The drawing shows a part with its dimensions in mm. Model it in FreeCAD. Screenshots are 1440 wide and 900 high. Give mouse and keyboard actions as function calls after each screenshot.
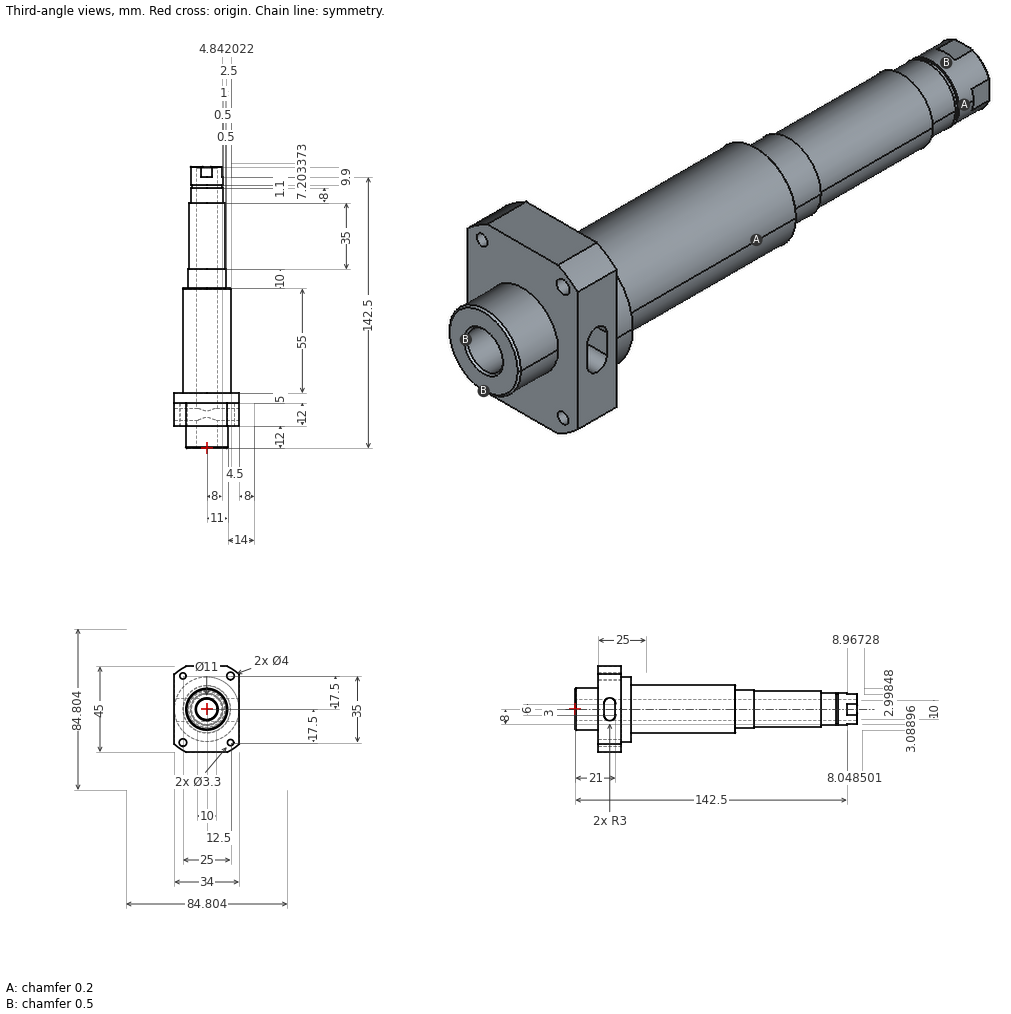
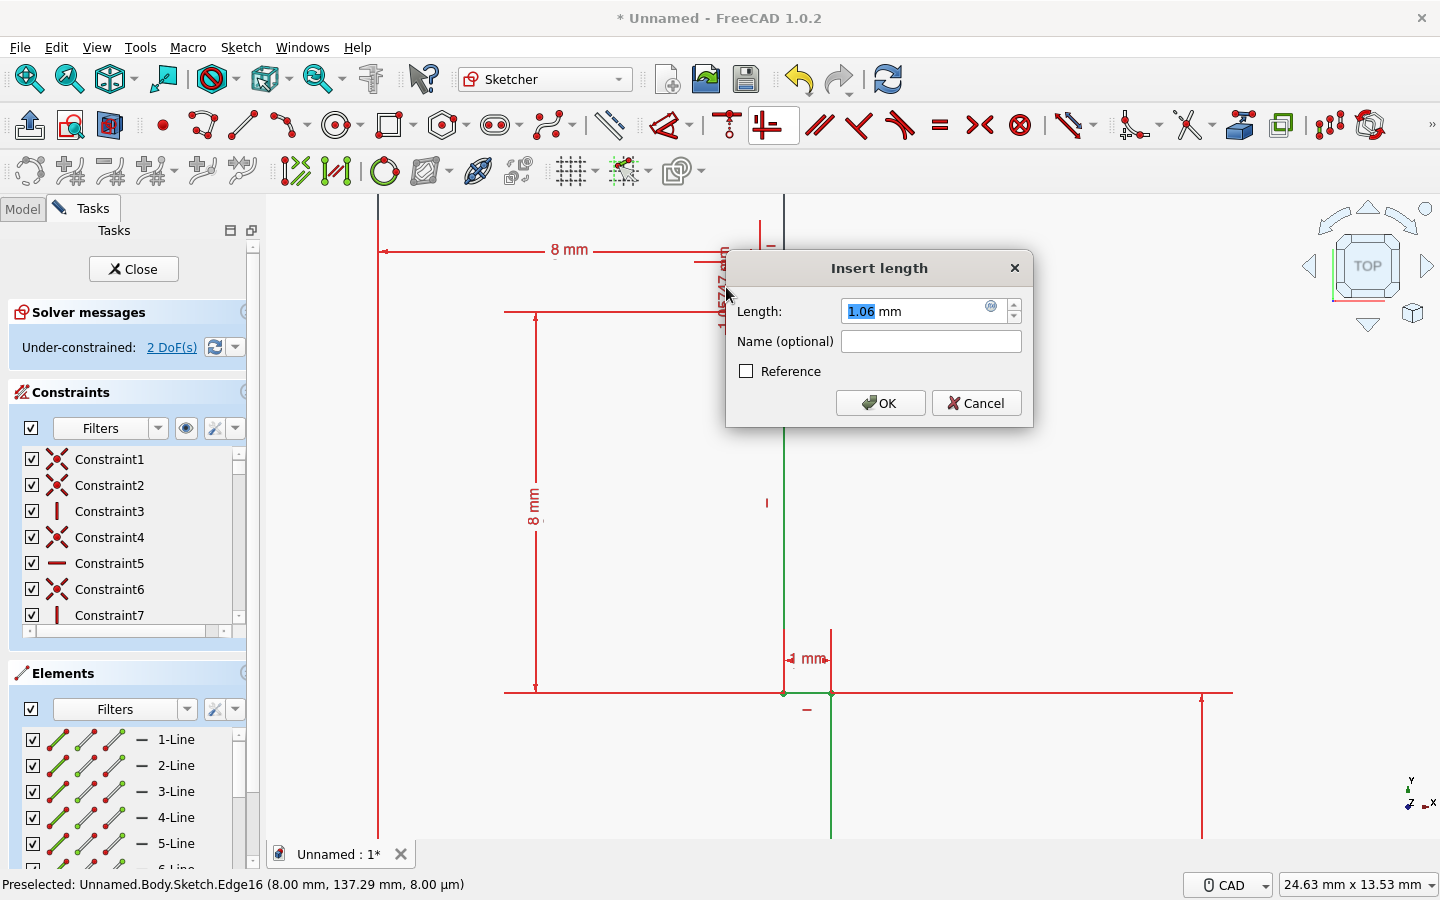
text(1.1)
key(Return)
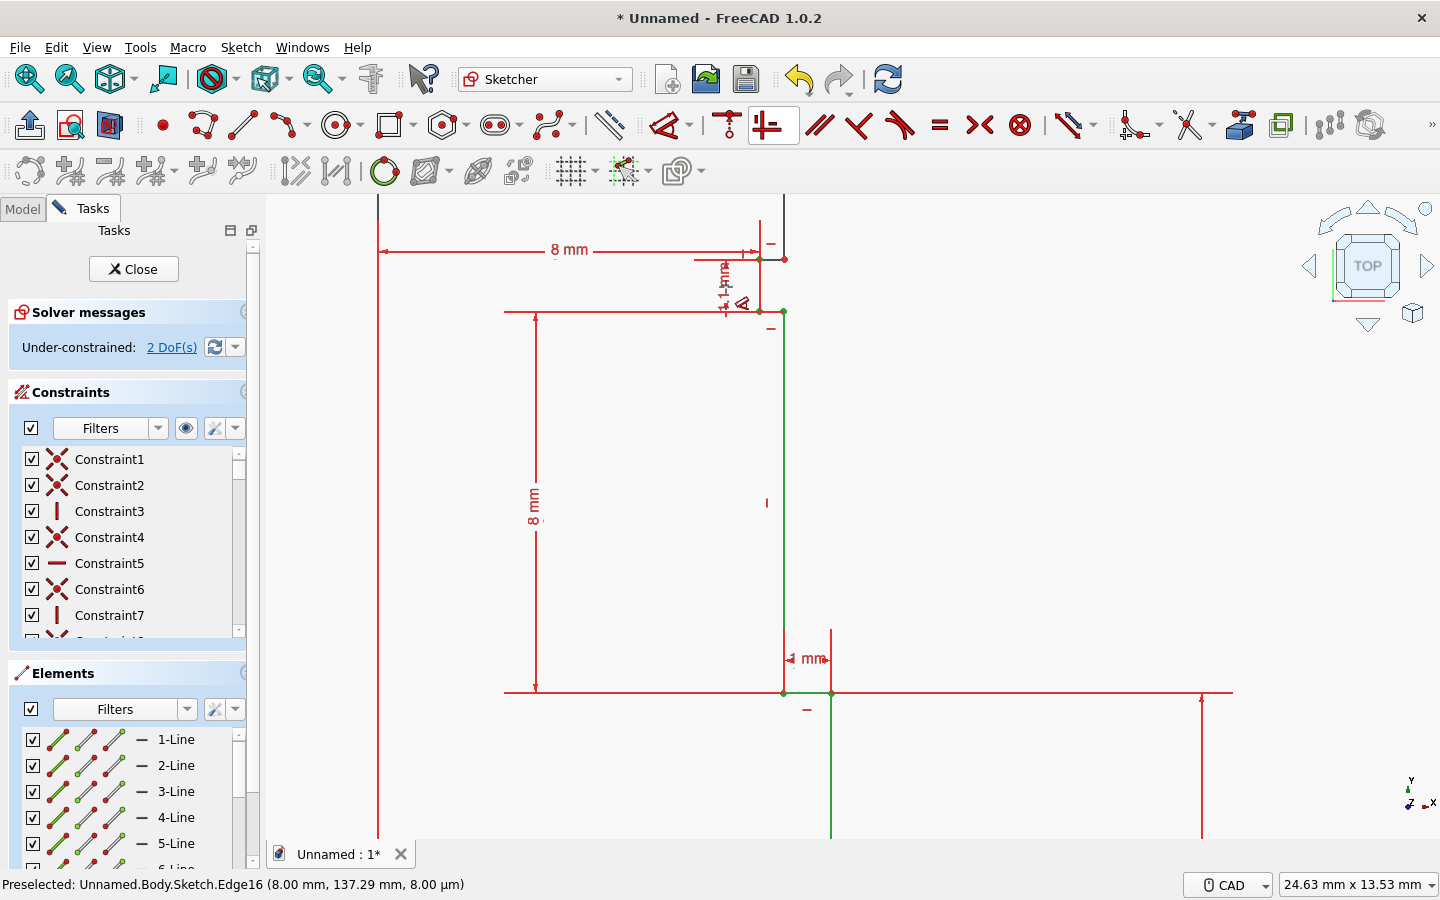
scroll(770, 260, up, 3)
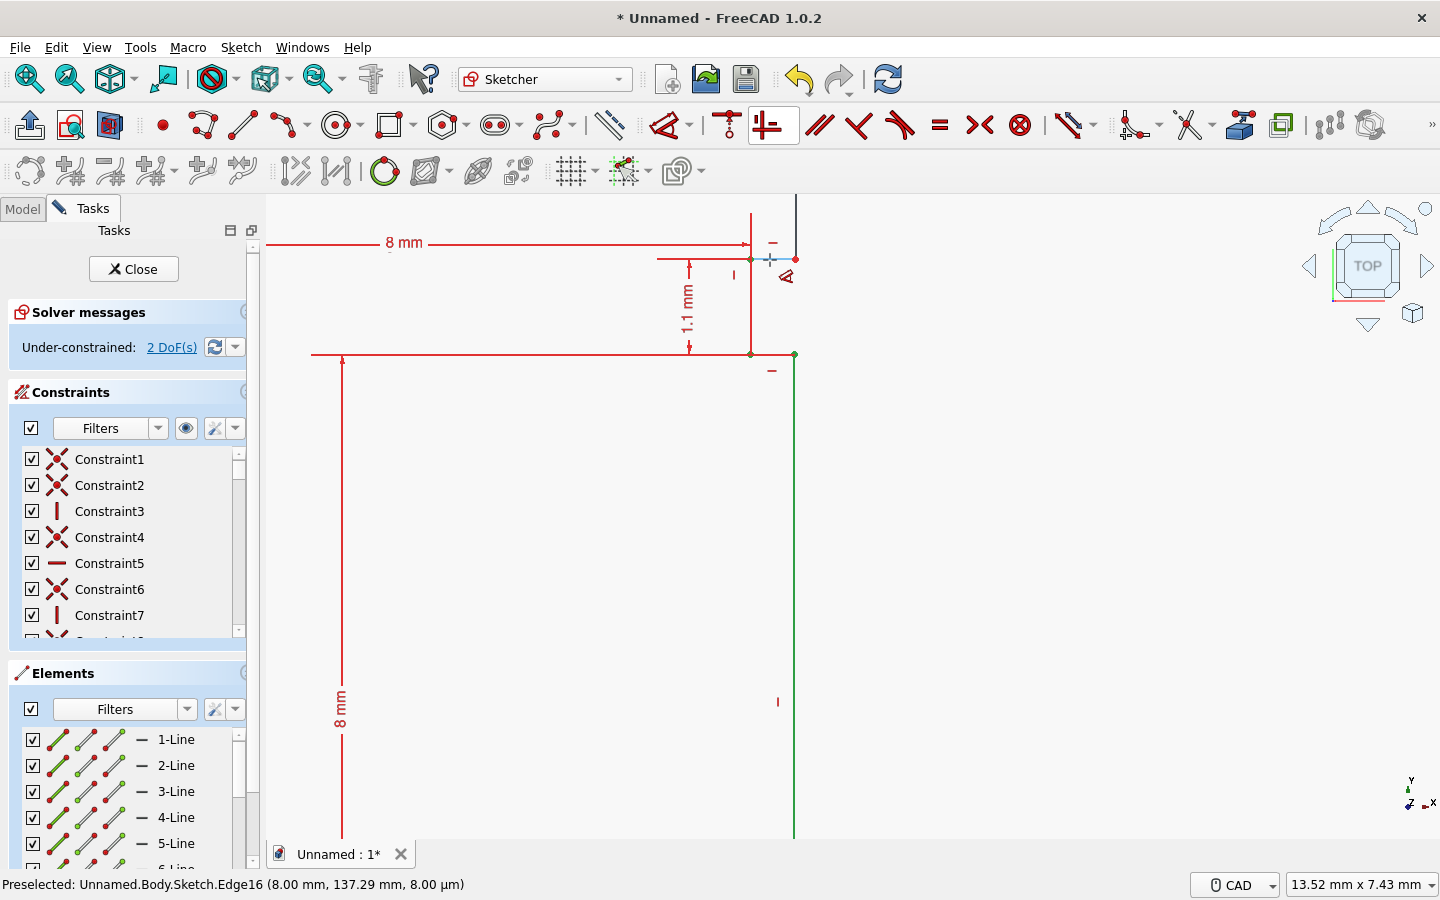
click(769, 259)
click(773, 225)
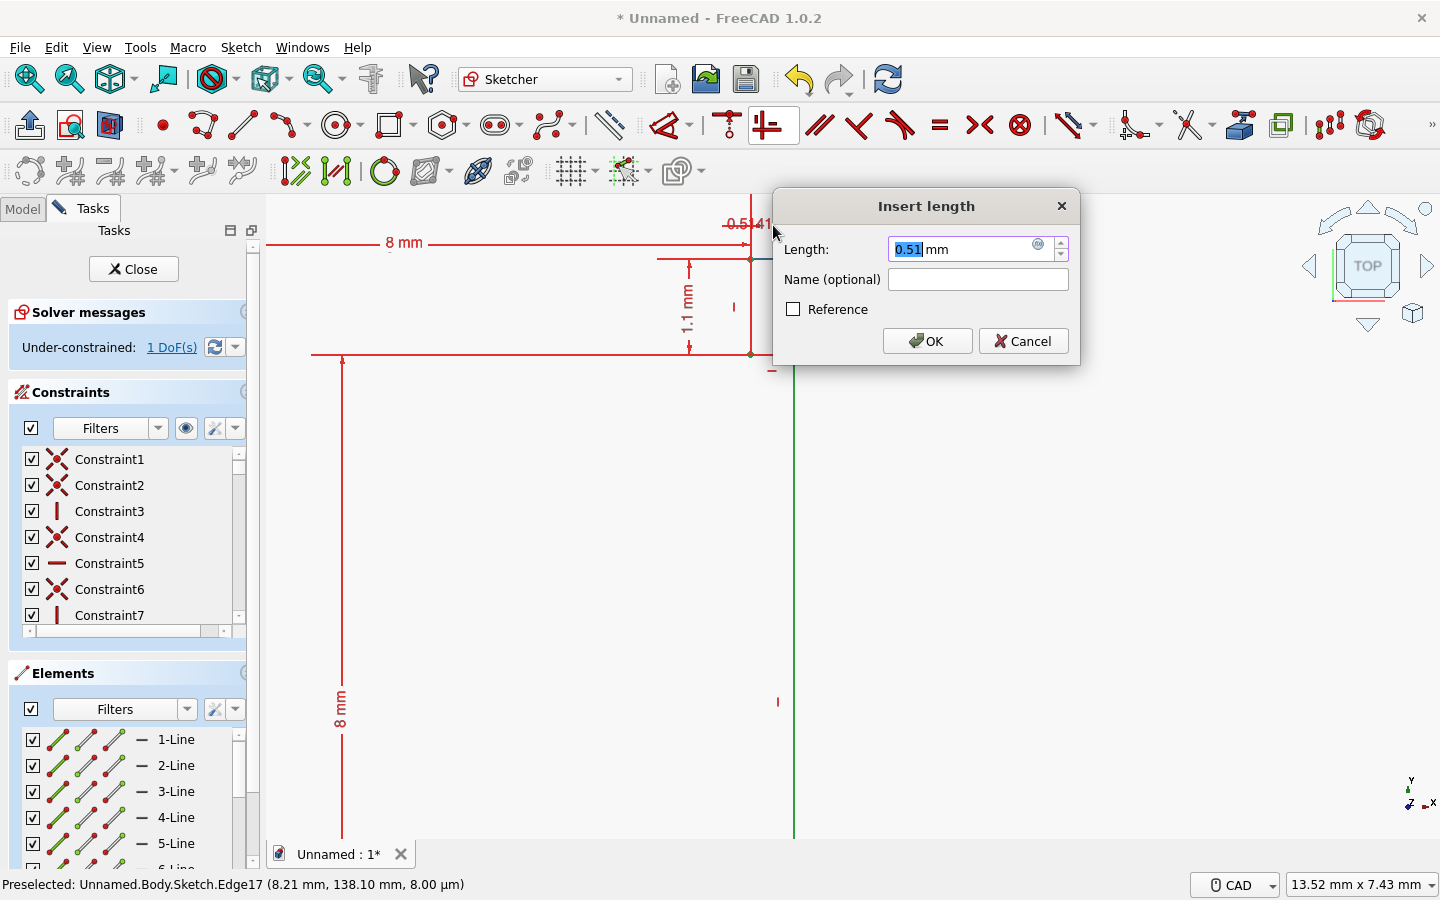
text(0.5)
key(Return)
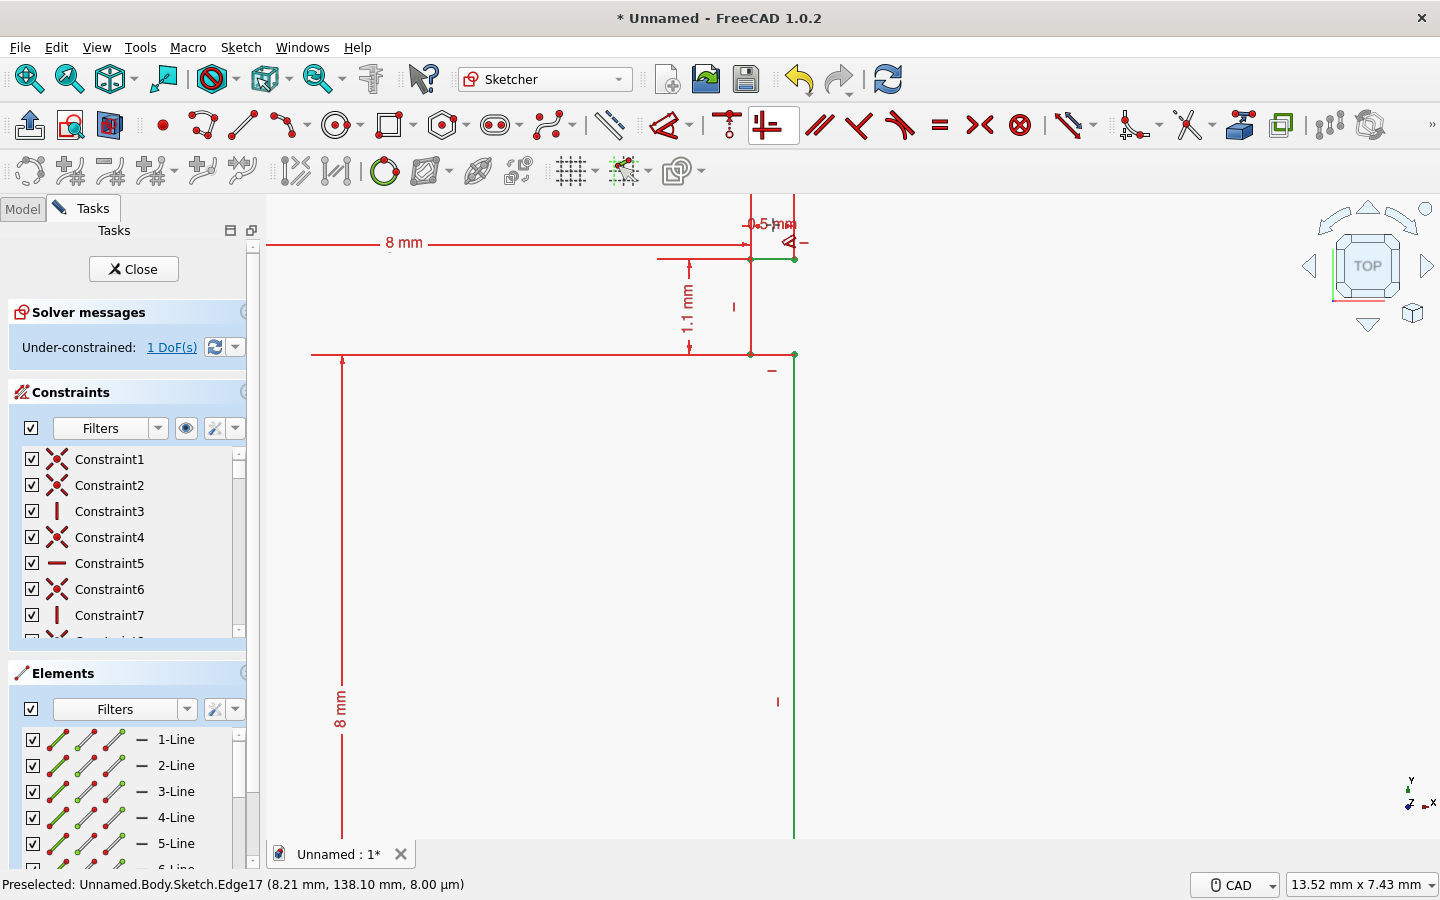
scroll(769, 291, down, 16)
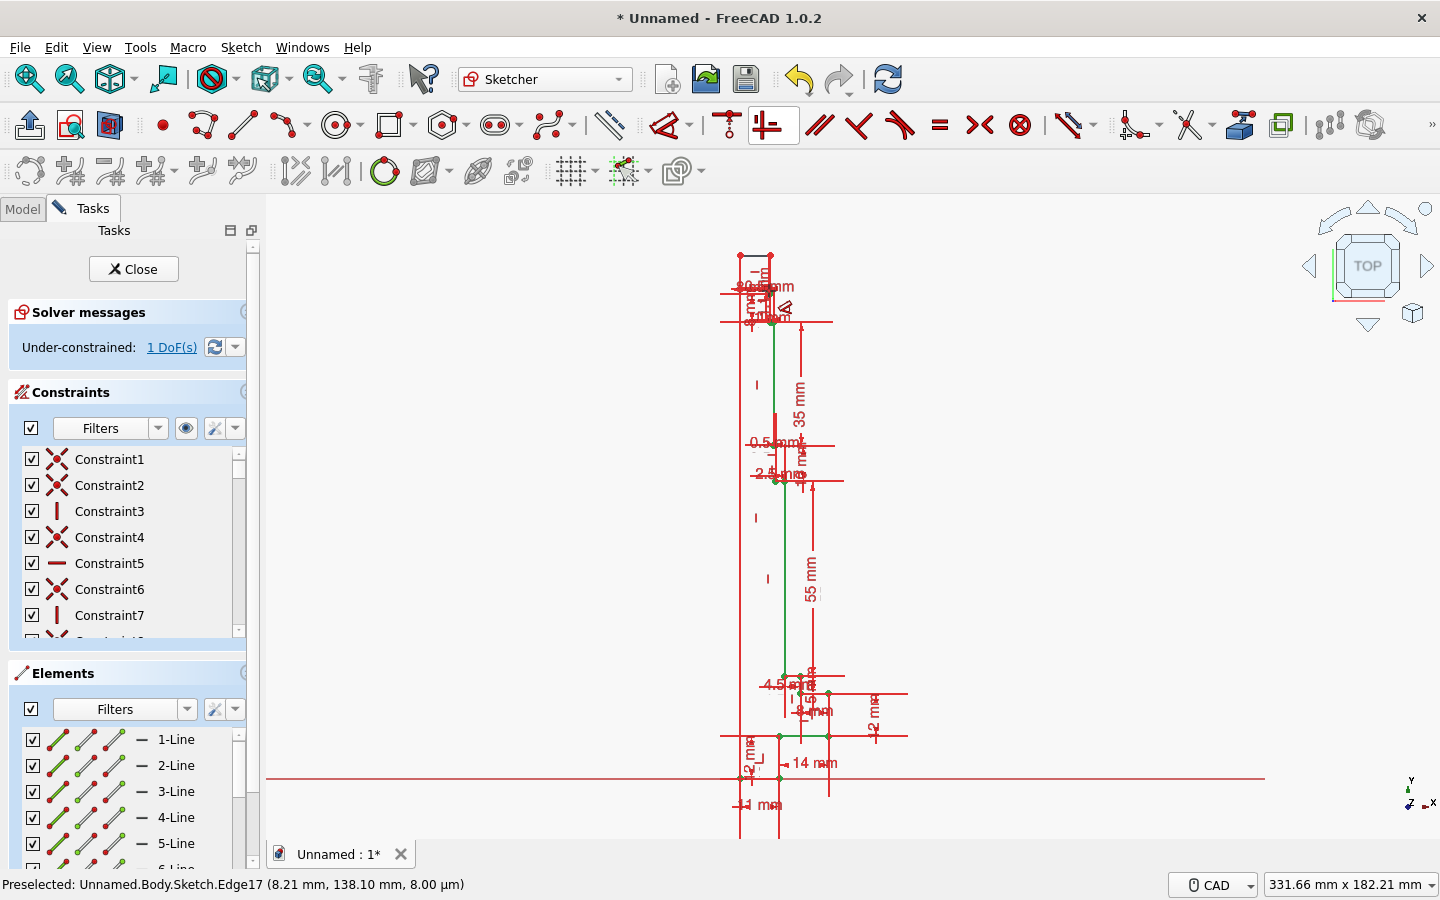
scroll(770, 280, up, 2)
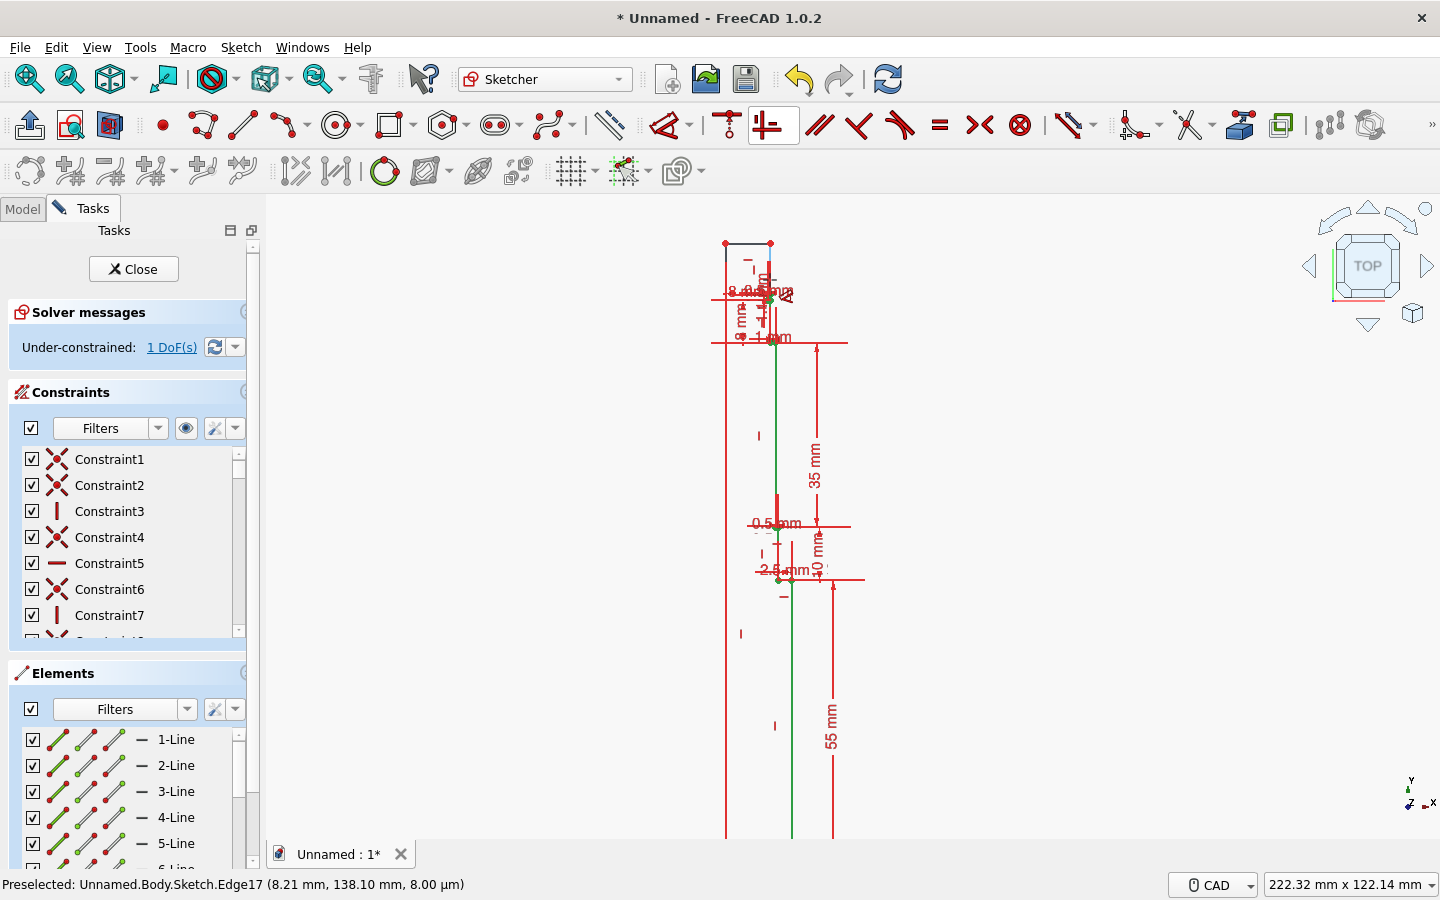
click(770, 279)
click(804, 269)